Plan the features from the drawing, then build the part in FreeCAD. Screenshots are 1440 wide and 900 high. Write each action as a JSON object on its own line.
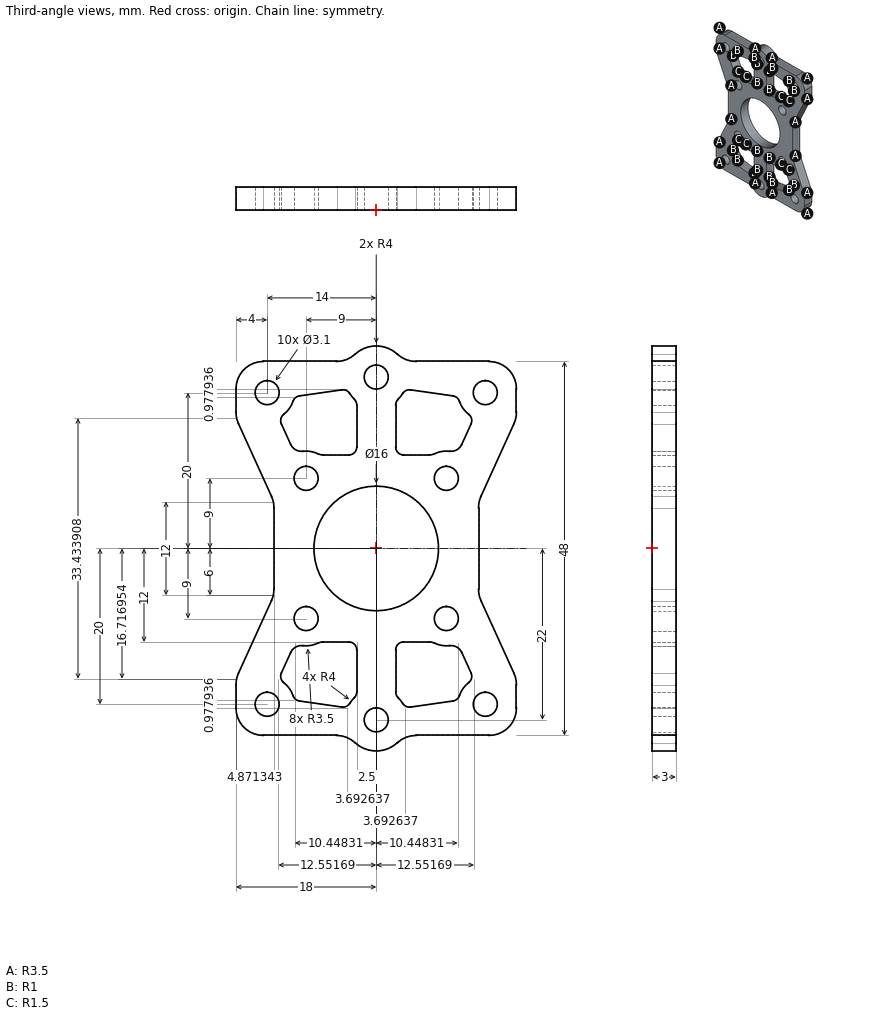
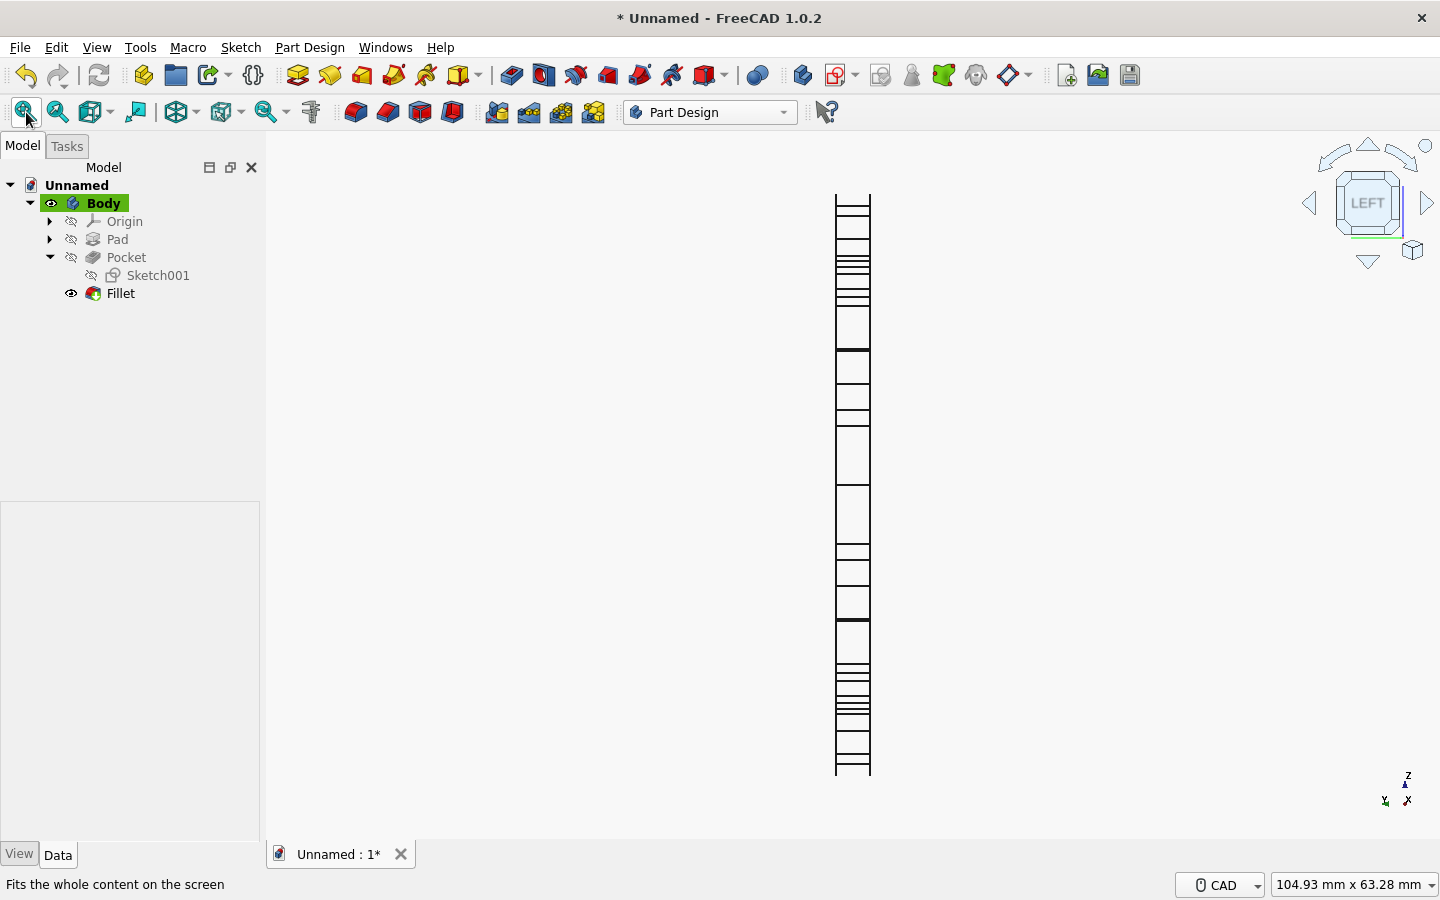
{"action": "key", "text": "0"}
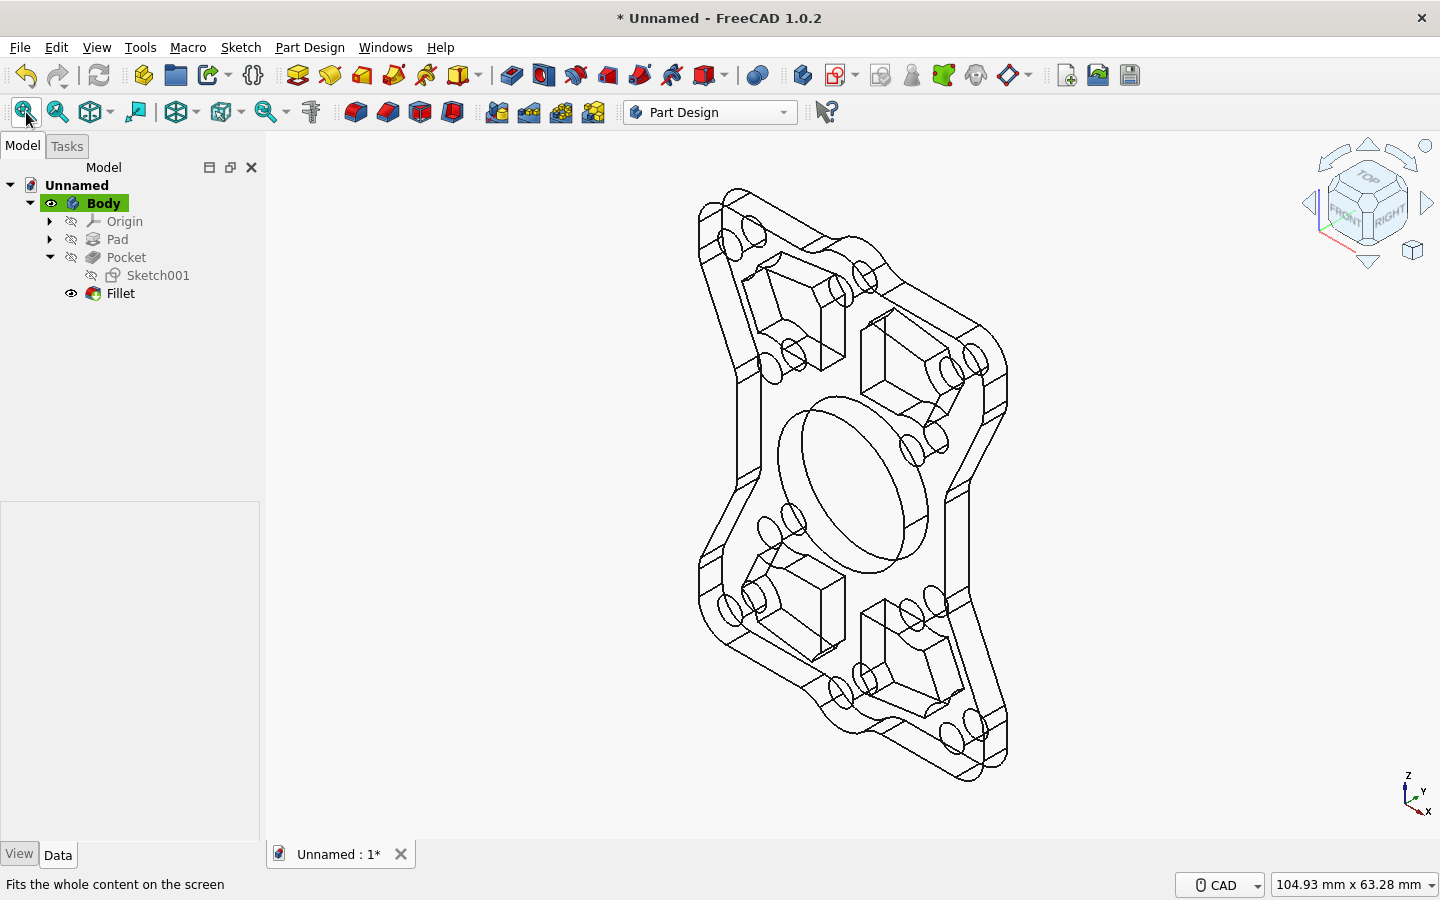
{"action": "left_click", "coordinate": [833, 363]}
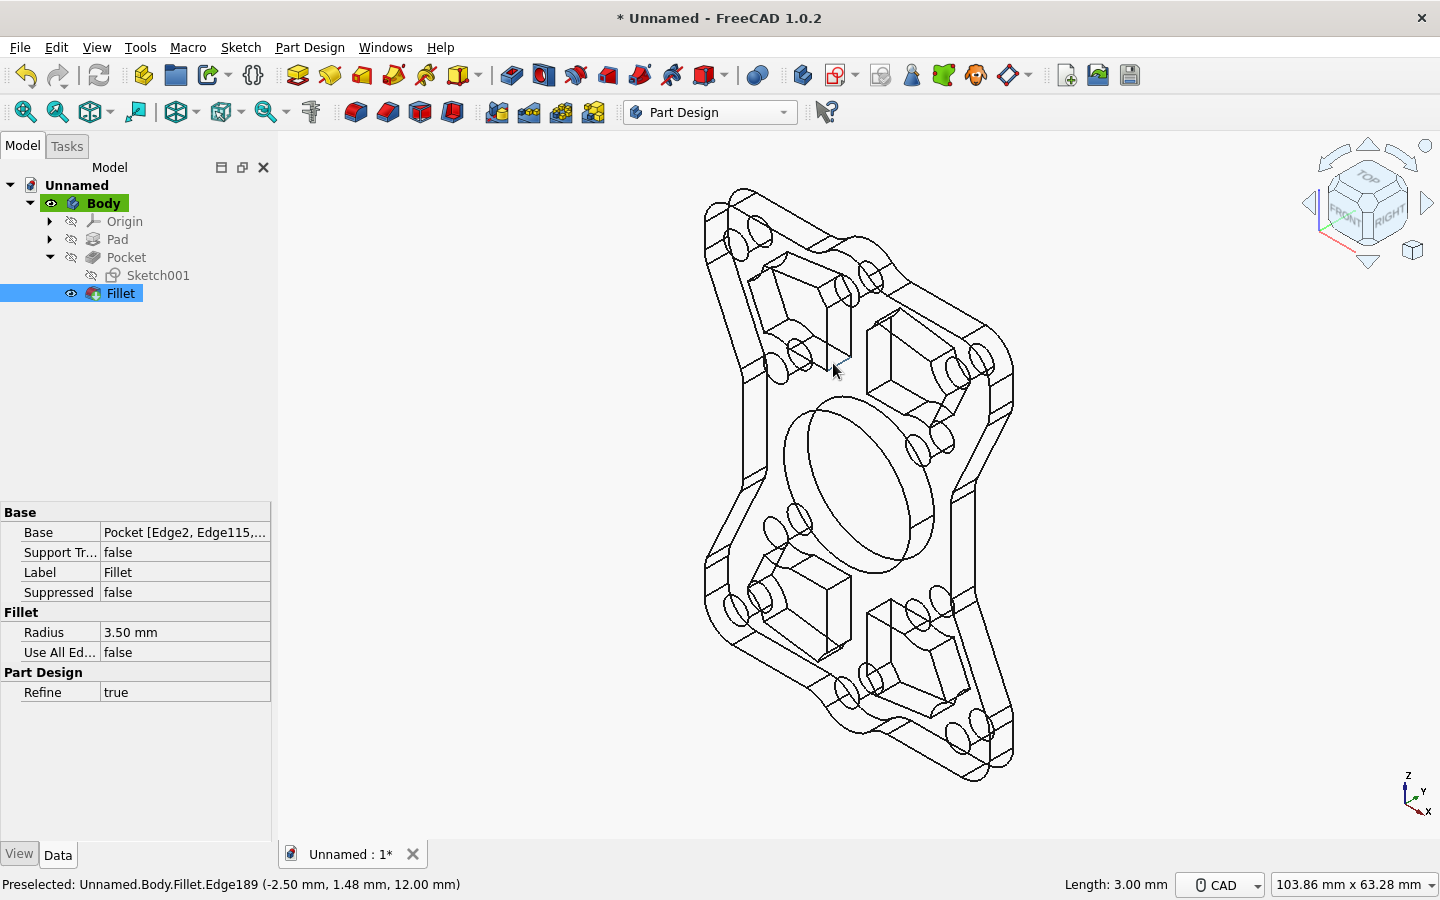
{"action": "left_click", "coordinate": [834, 303], "text": "ctrl"}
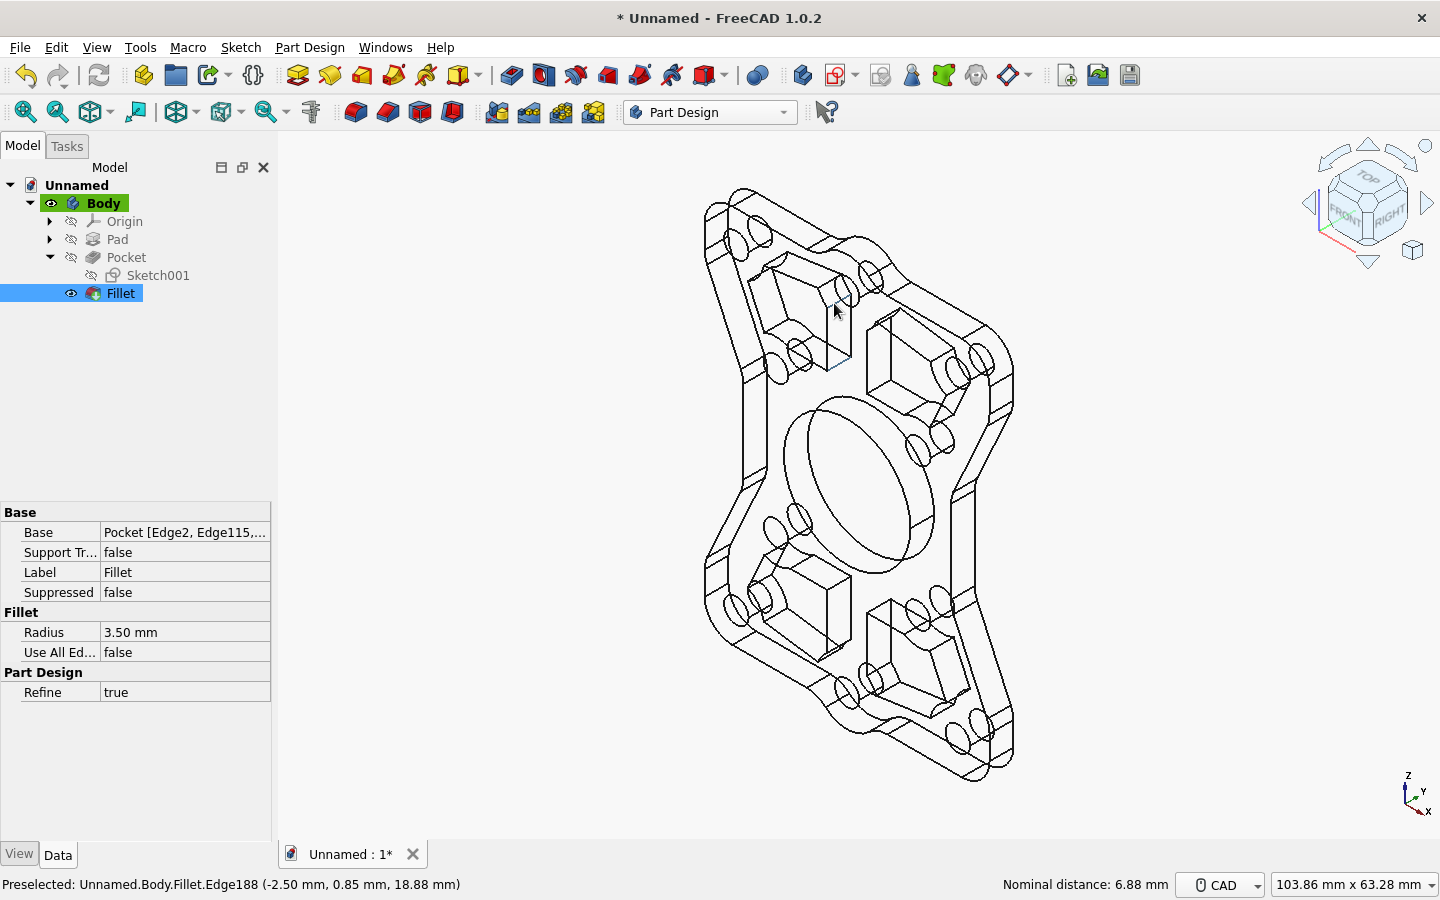
{"action": "left_click", "coordinate": [827, 282], "text": "ctrl"}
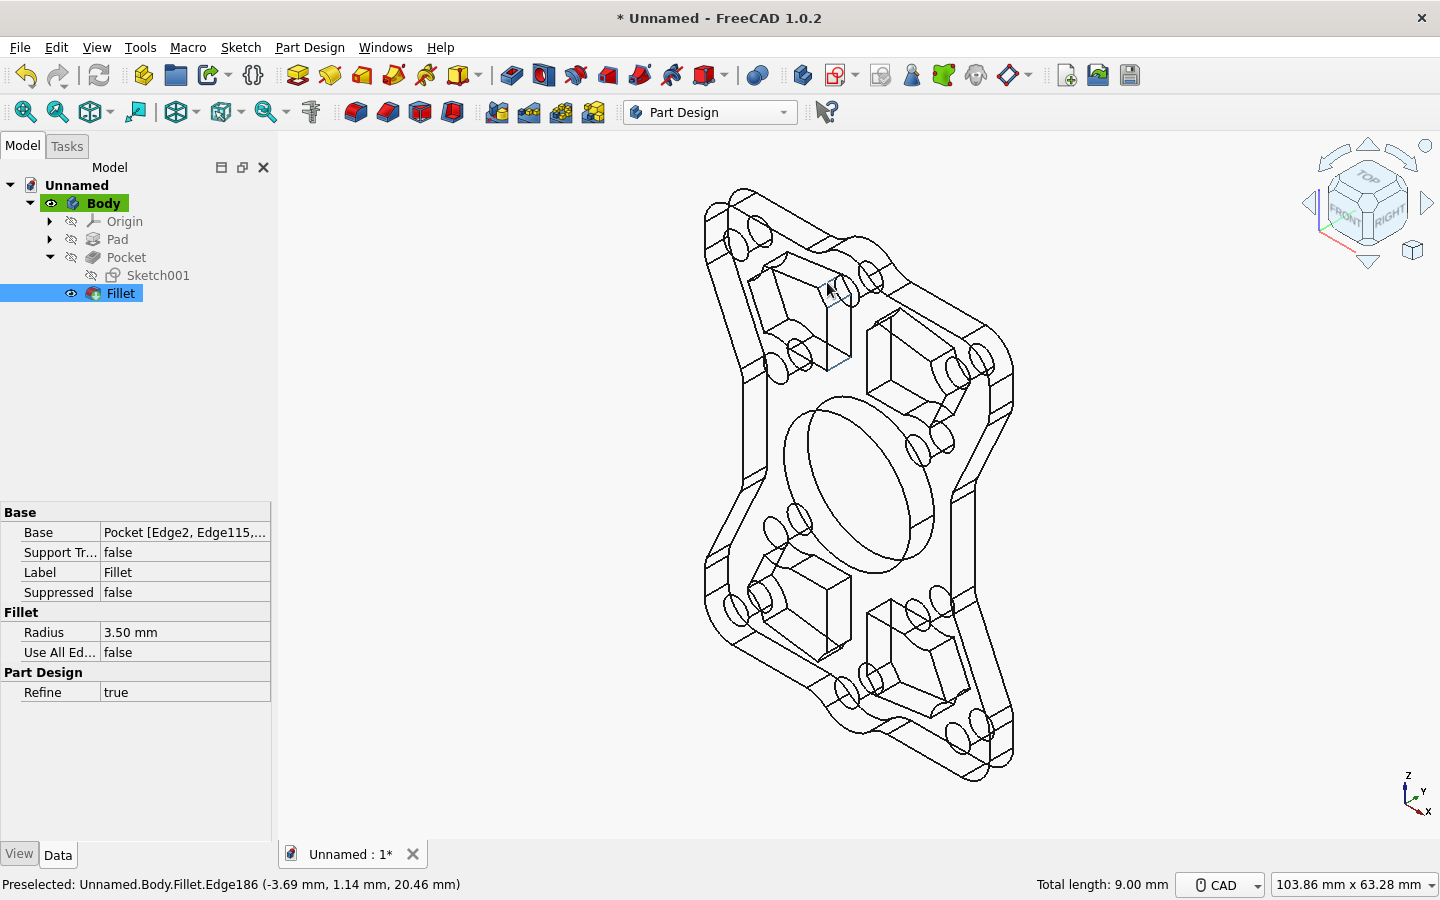
{"action": "left_click", "coordinate": [776, 258], "text": "ctrl"}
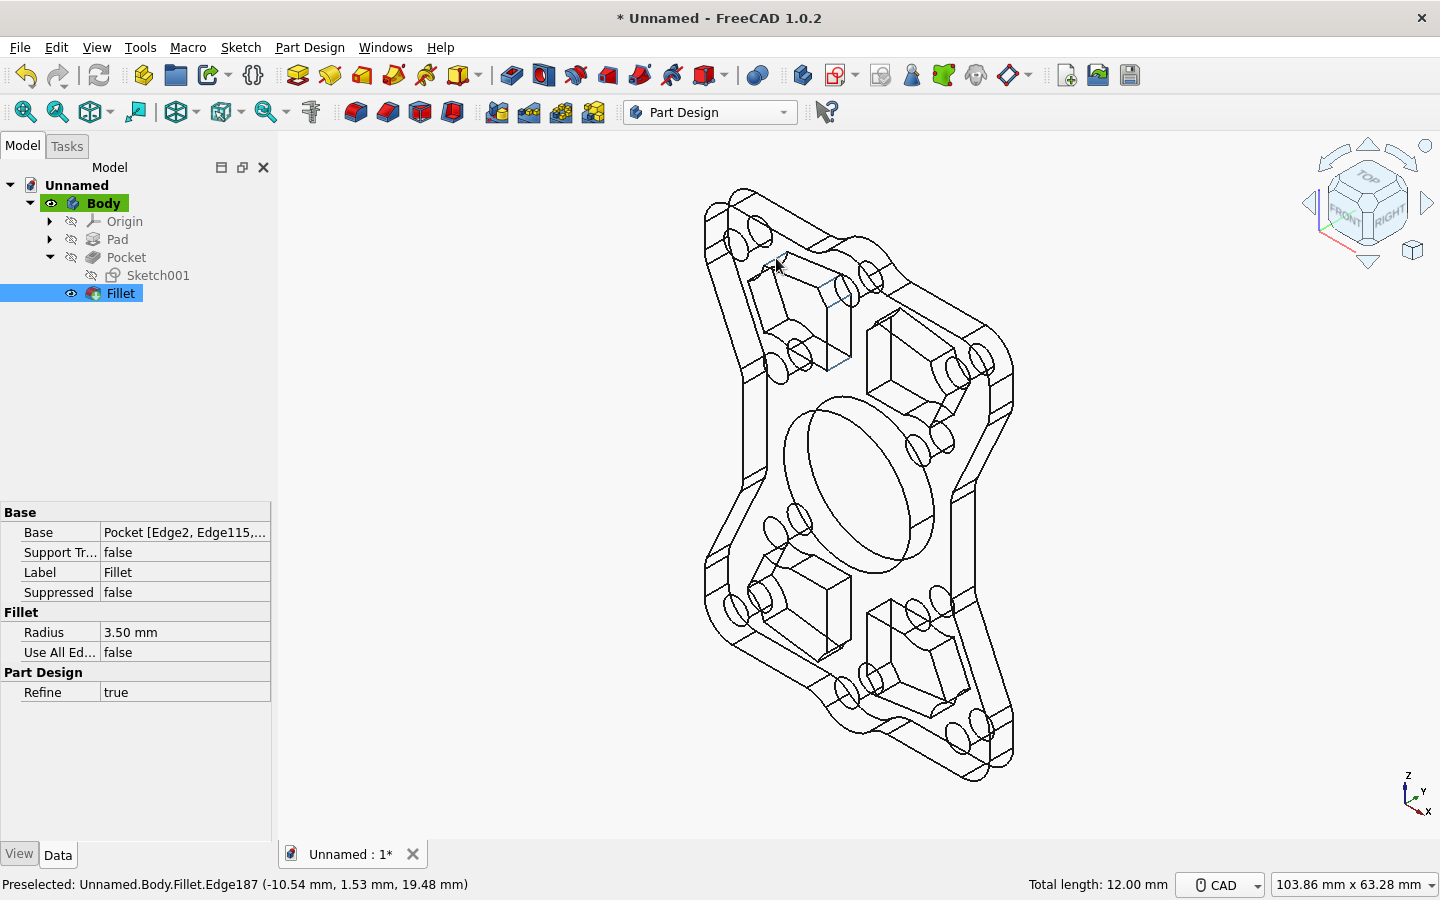
{"action": "left_click", "coordinate": [958, 695], "text": "ctrl"}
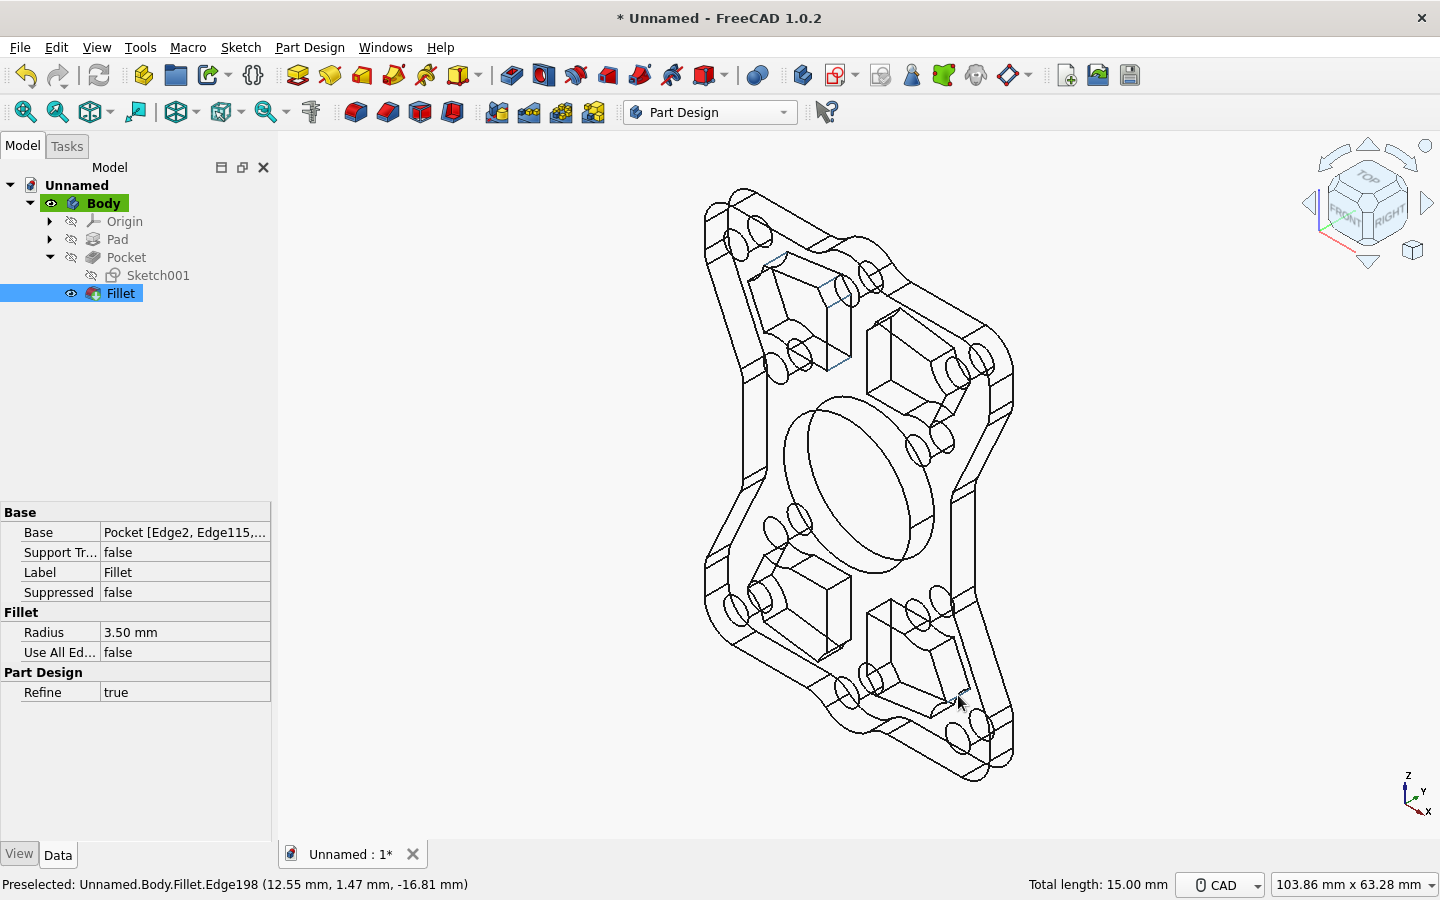
{"action": "left_click", "coordinate": [879, 605], "text": "ctrl"}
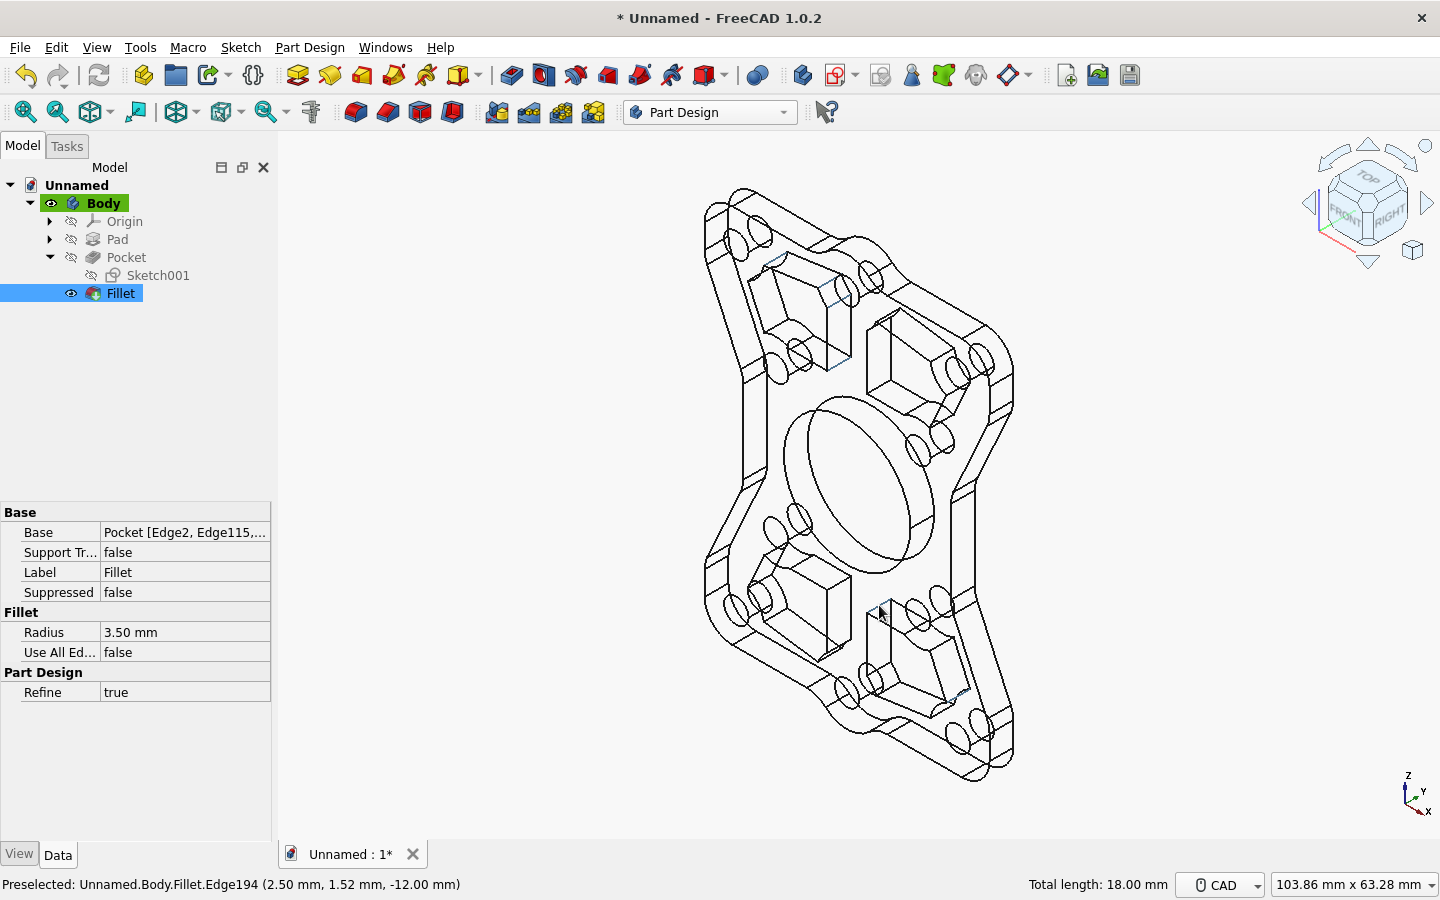
{"action": "left_click", "coordinate": [879, 668], "text": "ctrl"}